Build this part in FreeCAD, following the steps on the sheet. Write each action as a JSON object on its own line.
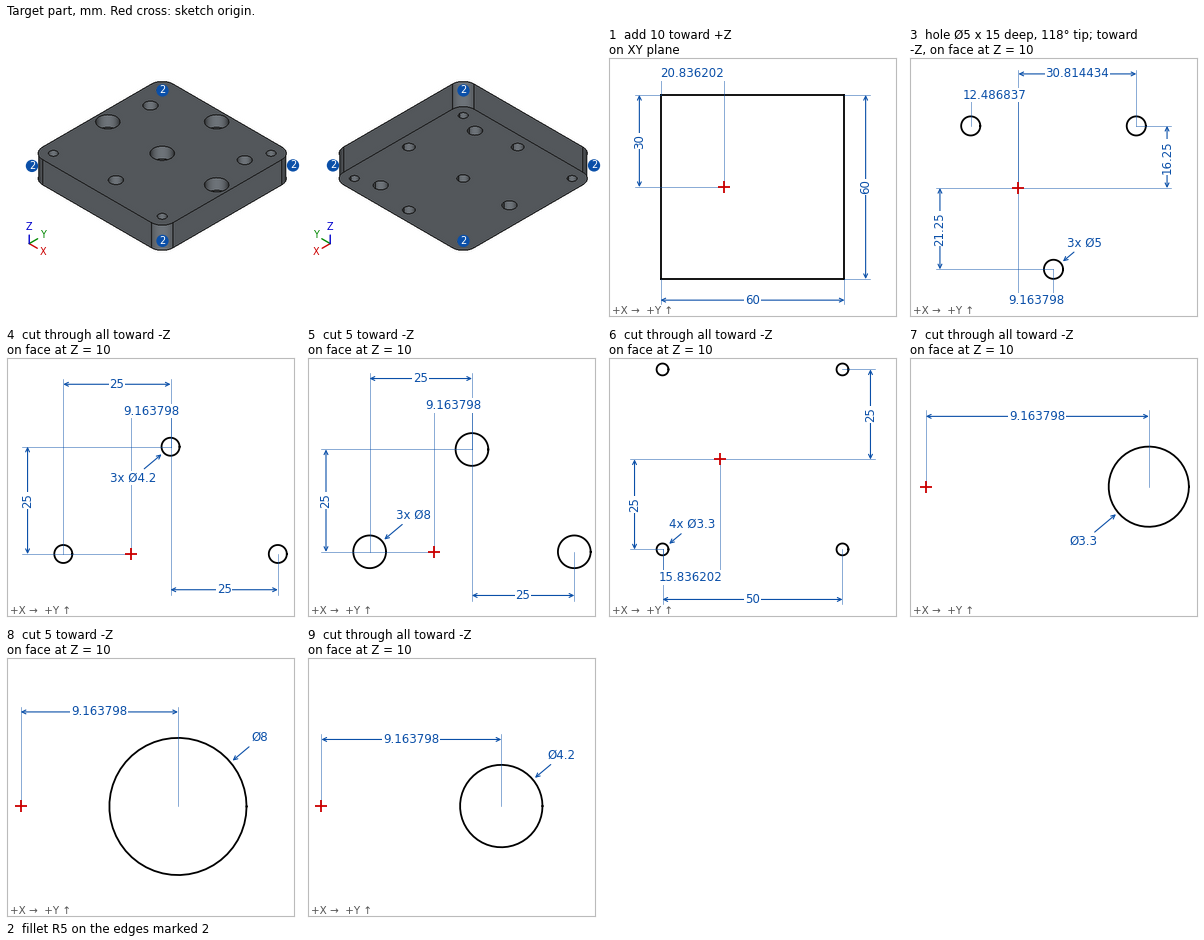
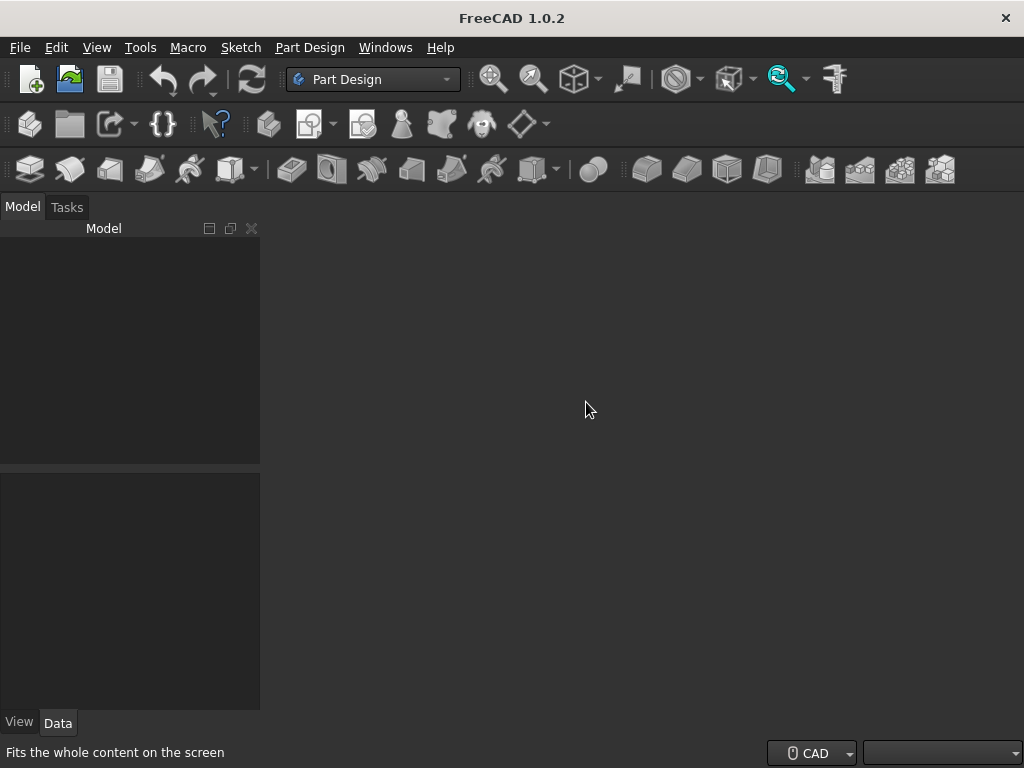
{"action": "left_click", "coordinate": [30, 80]}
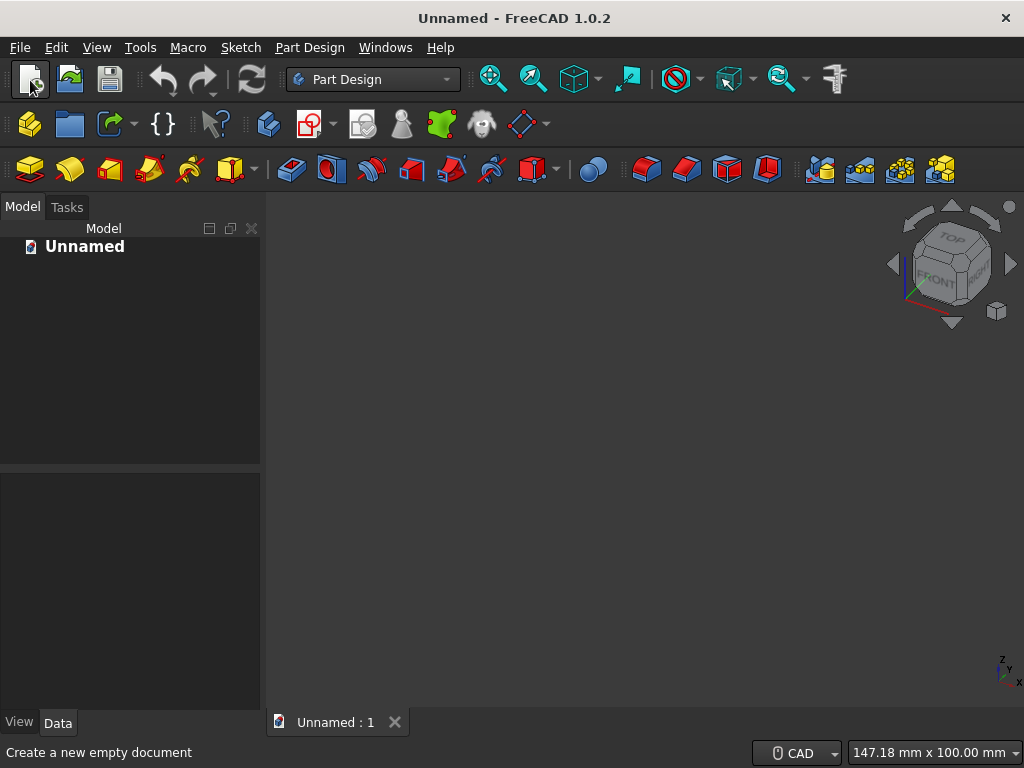
{"action": "left_click", "coordinate": [310, 124]}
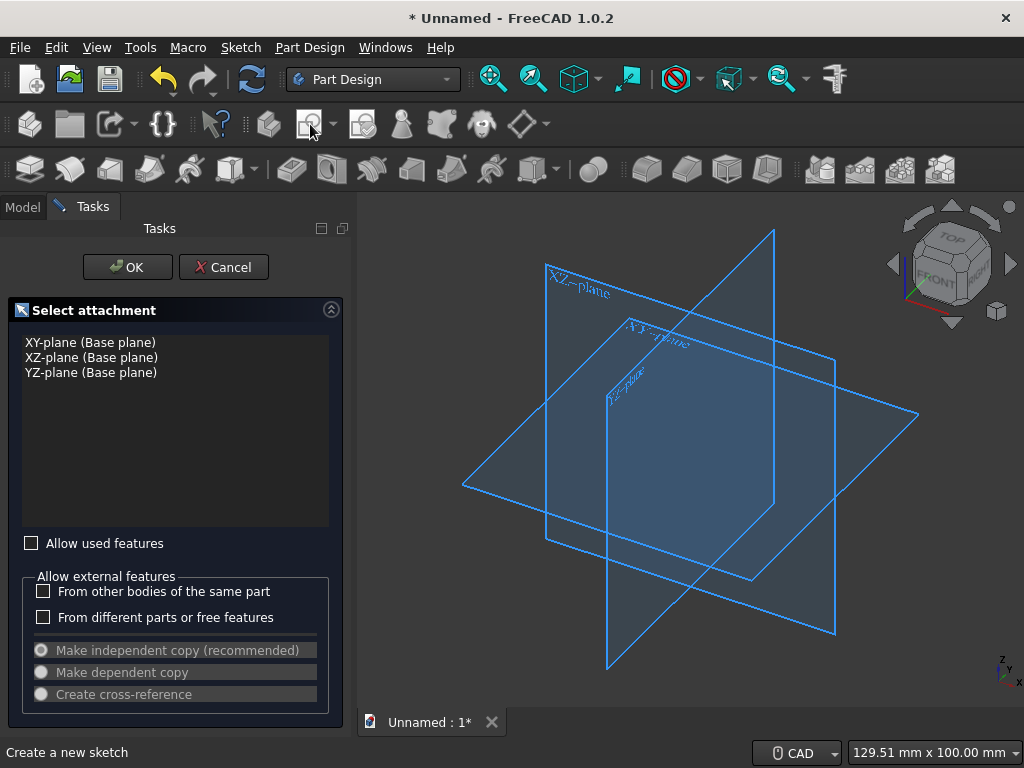
{"action": "left_click", "coordinate": [82, 342]}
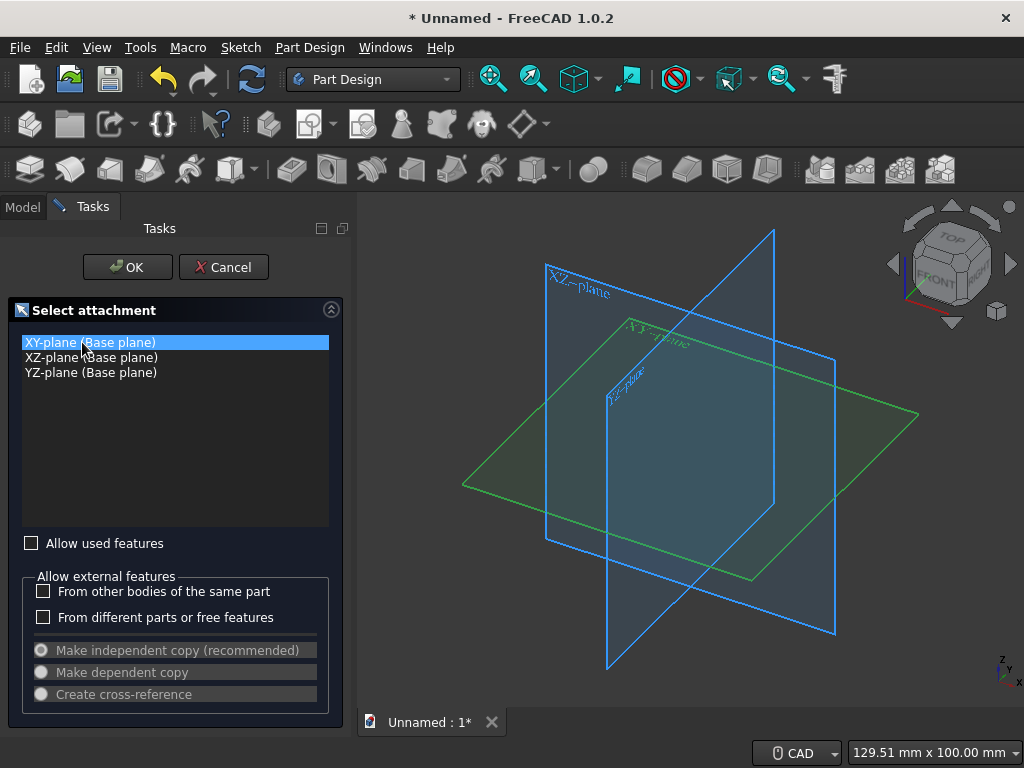
{"action": "left_click", "coordinate": [128, 267]}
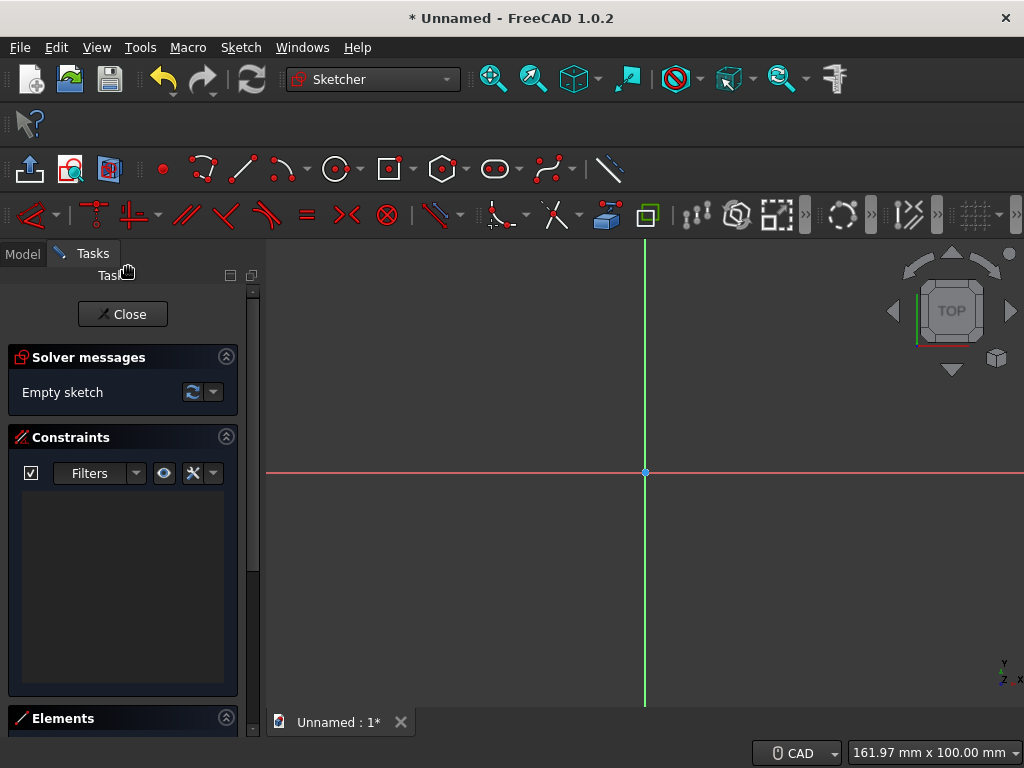
{"action": "key", "text": "g r"}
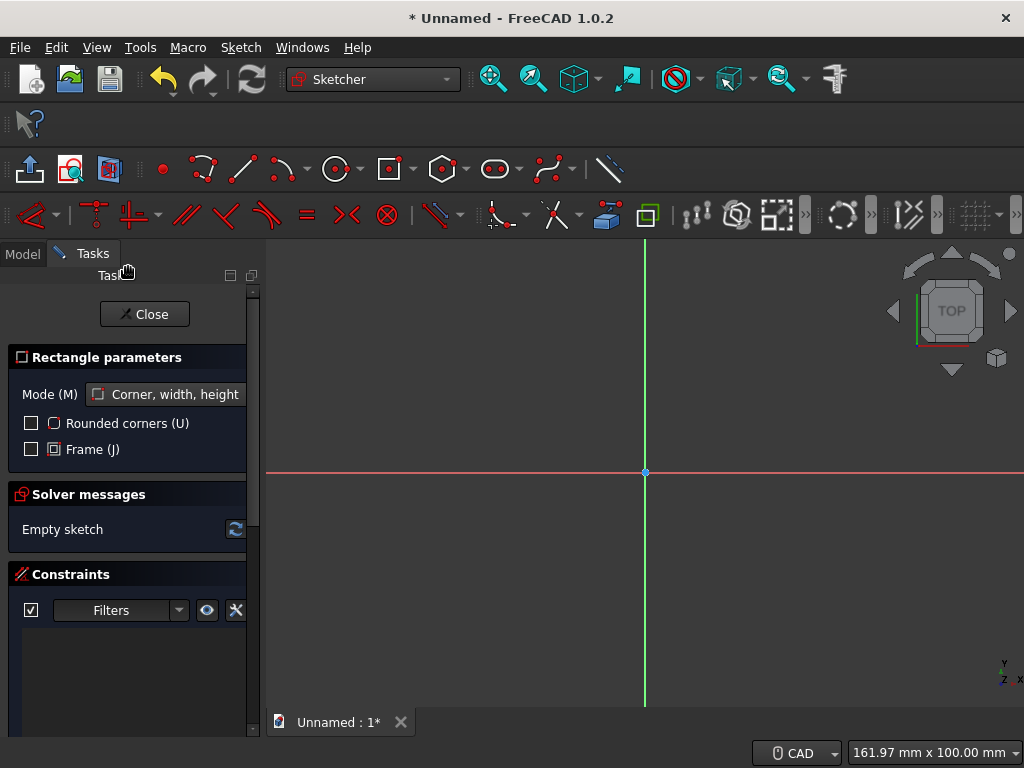
{"action": "left_click", "coordinate": [547, 333]}
{"action": "mouse_move", "coordinate": [828, 613]}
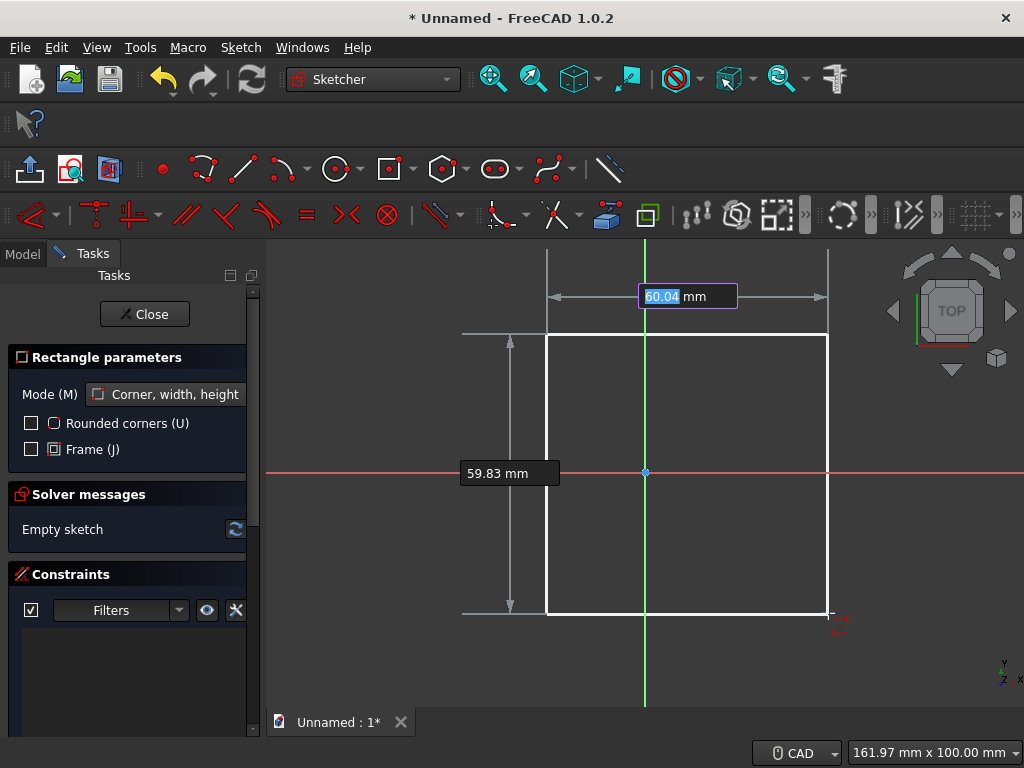
{"action": "type", "text": "60"}
{"action": "key", "text": "Tab"}
{"action": "type", "text": "60"}
{"action": "key", "text": "Return"}
{"action": "key", "text": "Escape"}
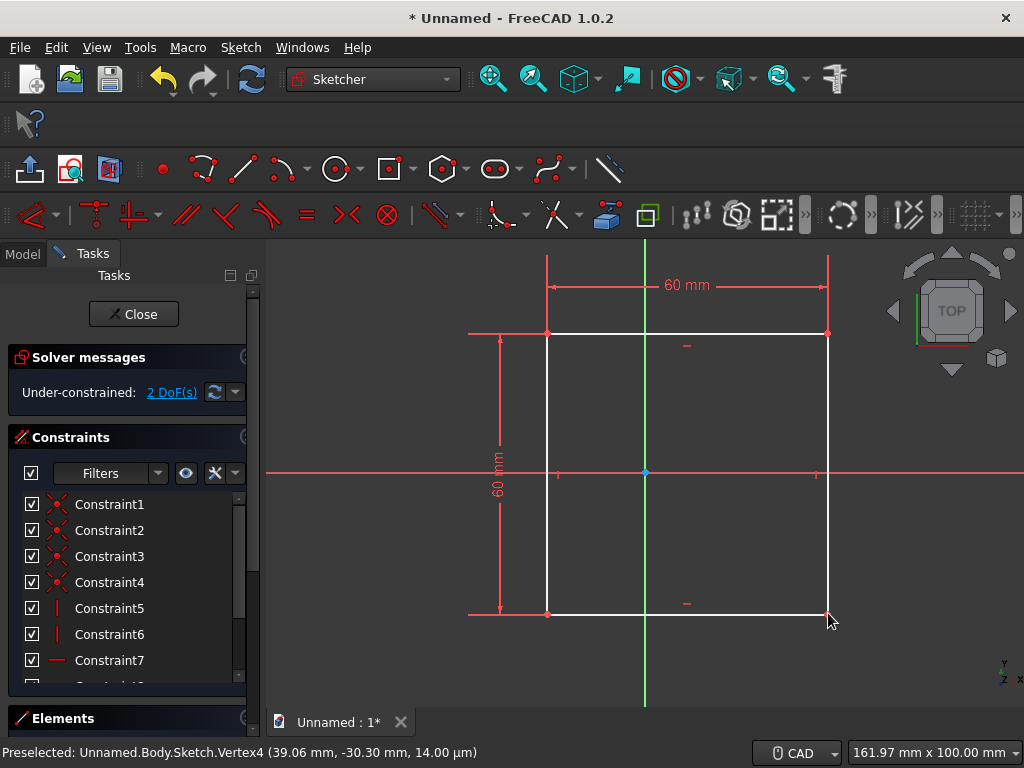
{"action": "left_click", "coordinate": [32, 216]}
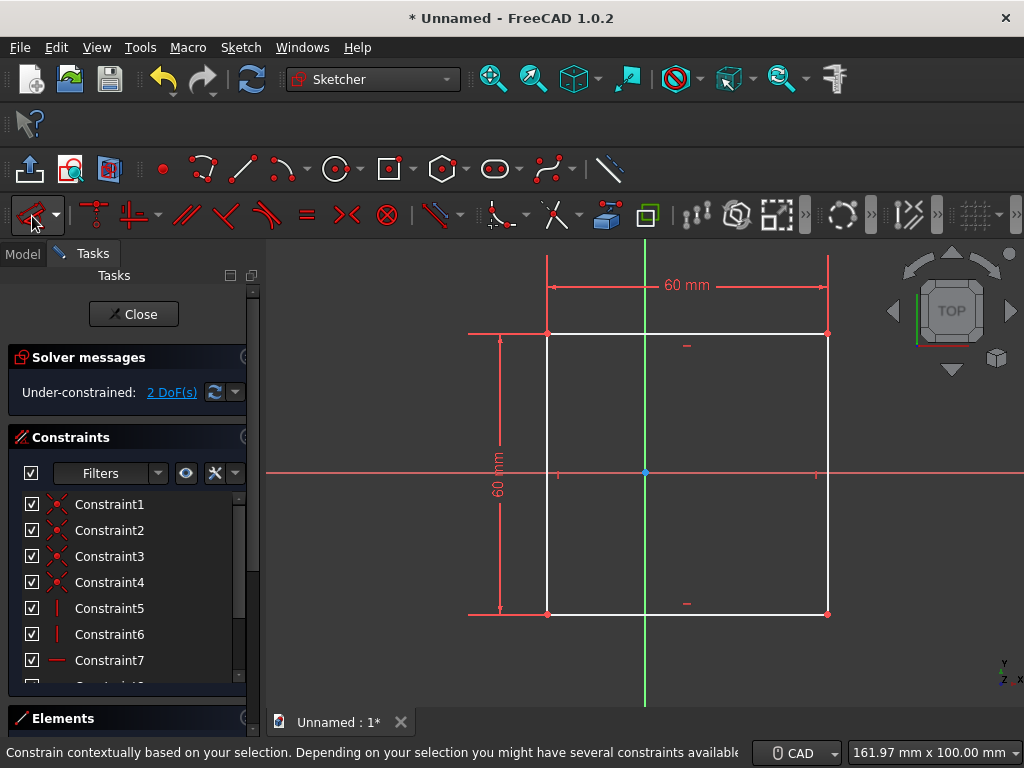
{"action": "left_click", "coordinate": [547, 334]}
{"action": "left_click", "coordinate": [513, 403]}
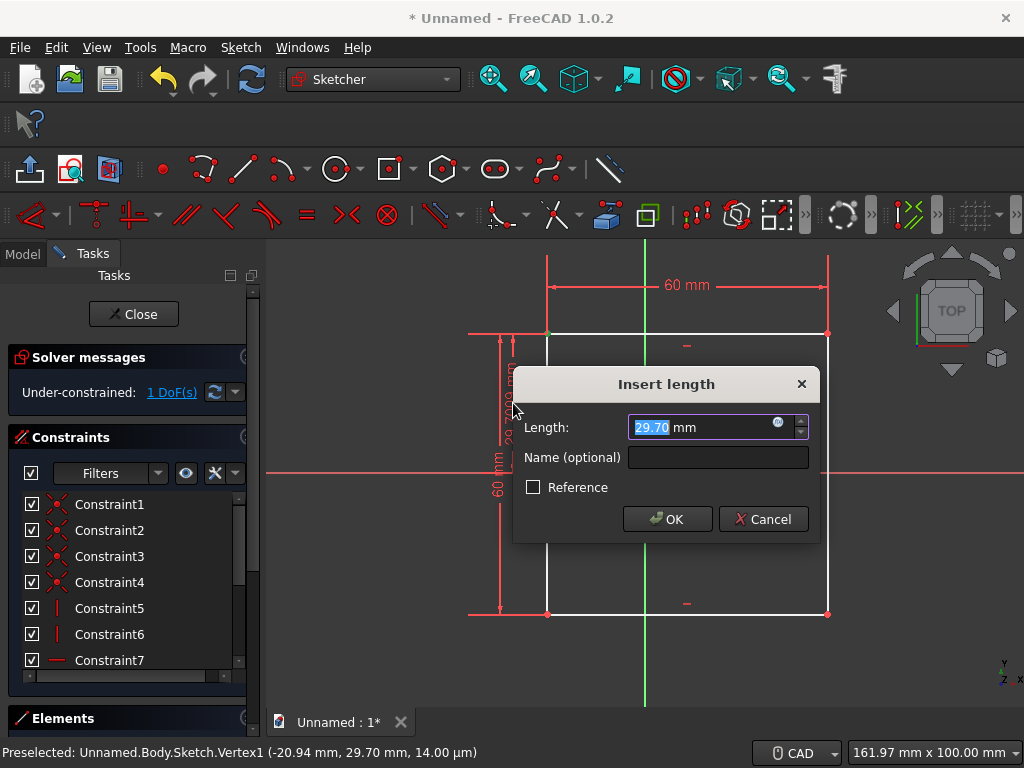
{"action": "type", "text": "30"}
{"action": "key", "text": "Return"}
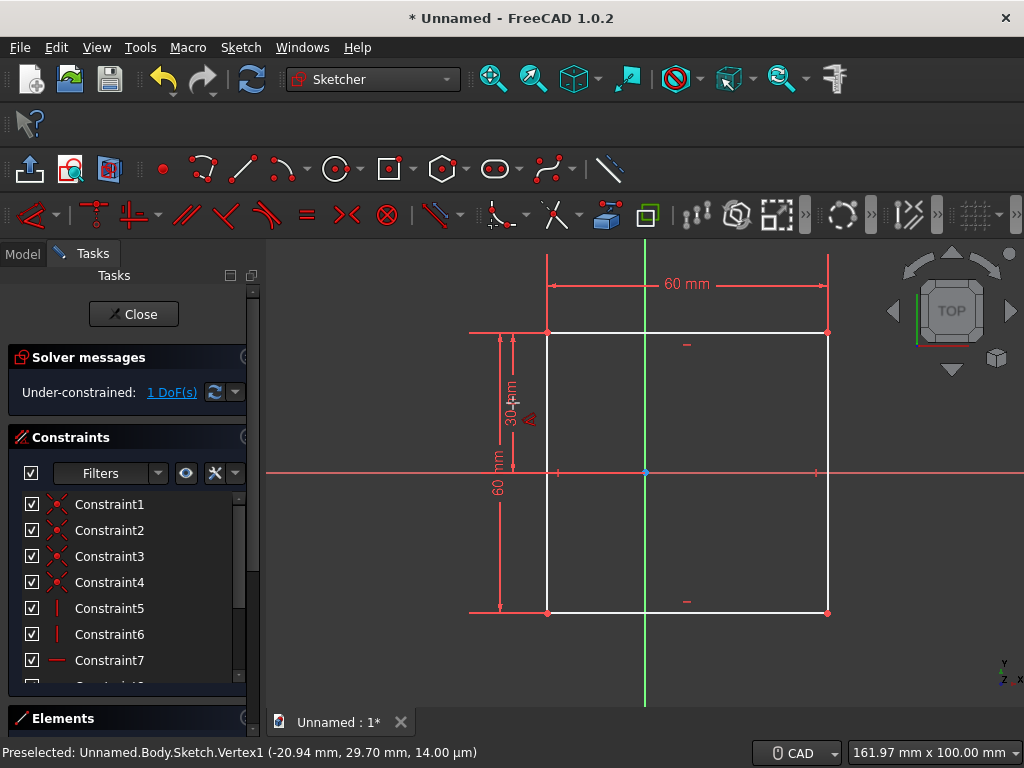
{"action": "left_click", "coordinate": [547, 333]}
{"action": "left_click", "coordinate": [596, 299]}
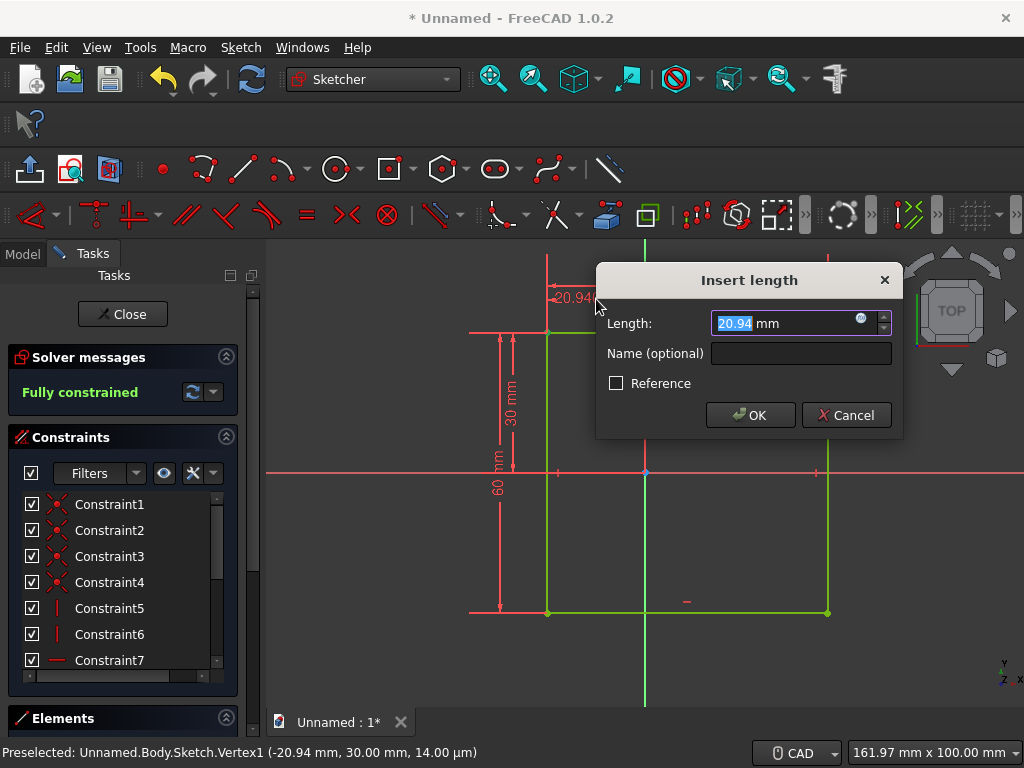
{"action": "type", "text": "20.836202"}
{"action": "key", "text": "Return"}
{"action": "key", "text": "Escape"}